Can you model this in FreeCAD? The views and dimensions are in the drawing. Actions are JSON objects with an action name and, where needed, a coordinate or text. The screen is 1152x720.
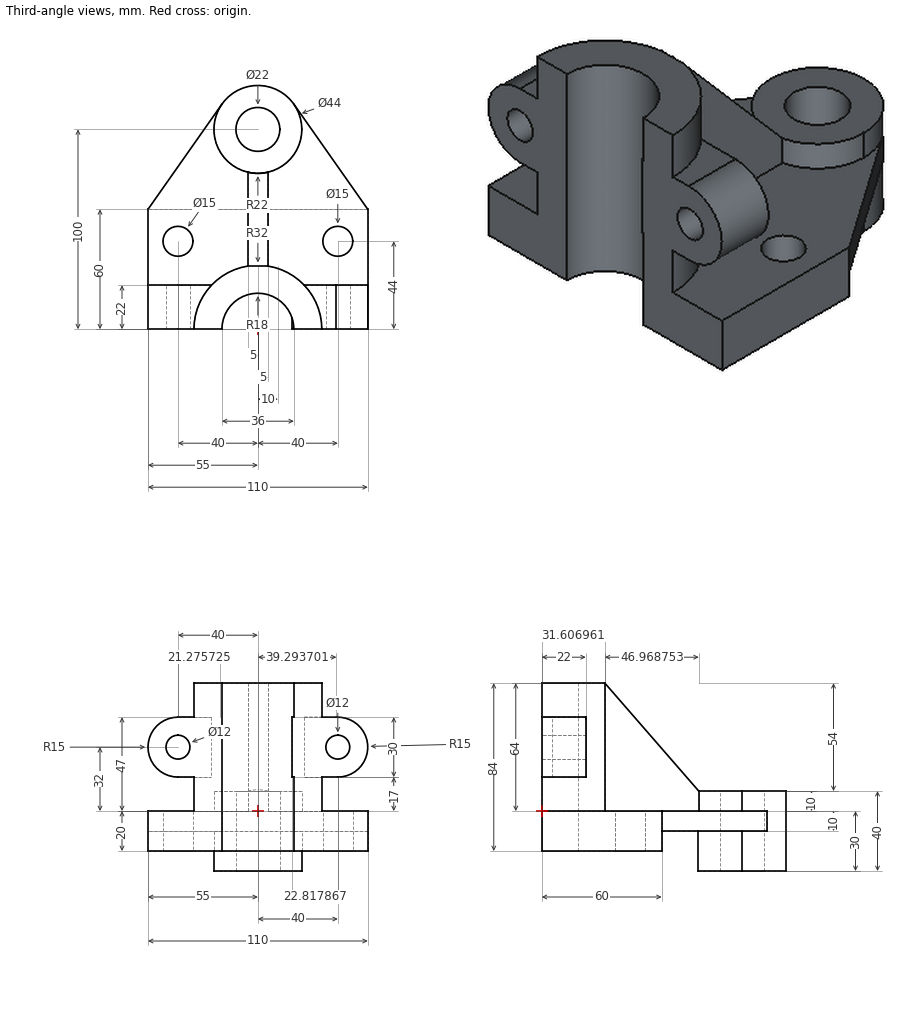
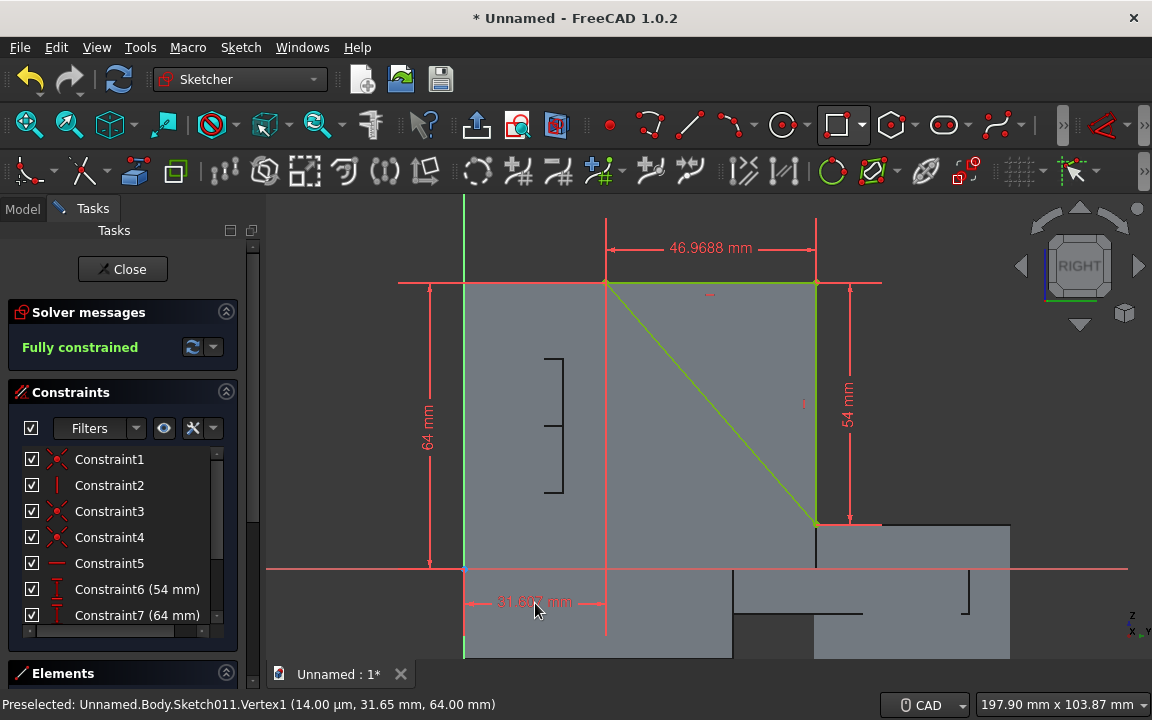
{"action": "left_click", "coordinate": [123, 269]}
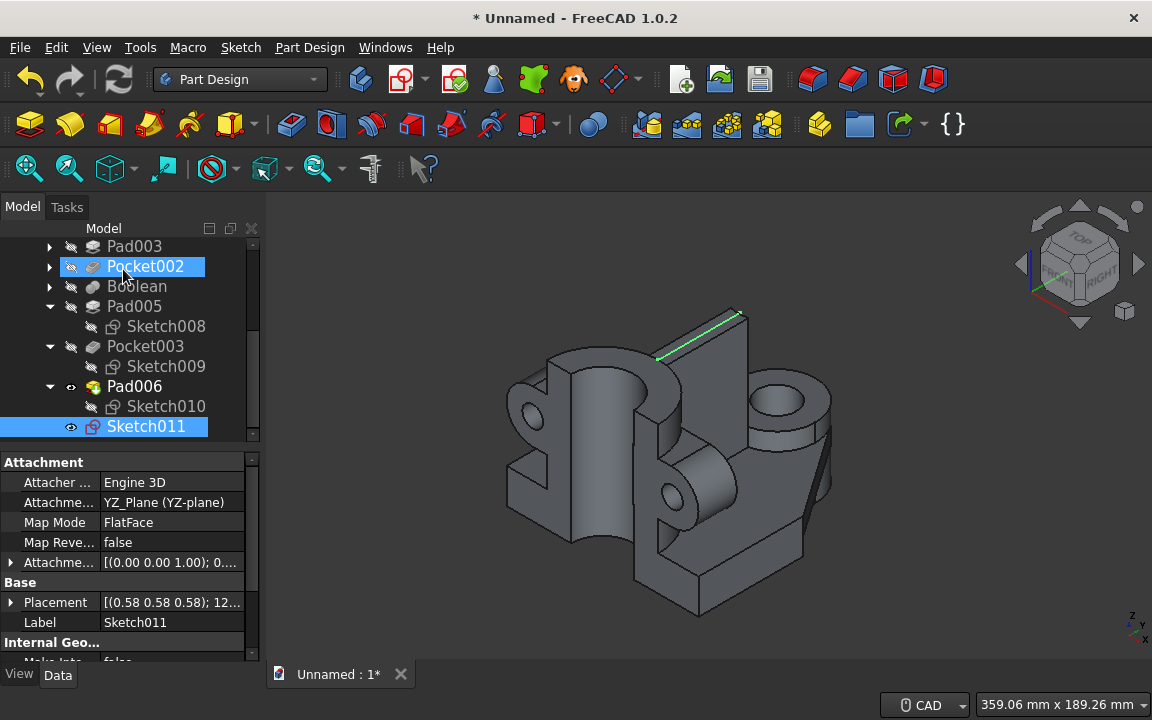
{"action": "left_click", "coordinate": [292, 124]}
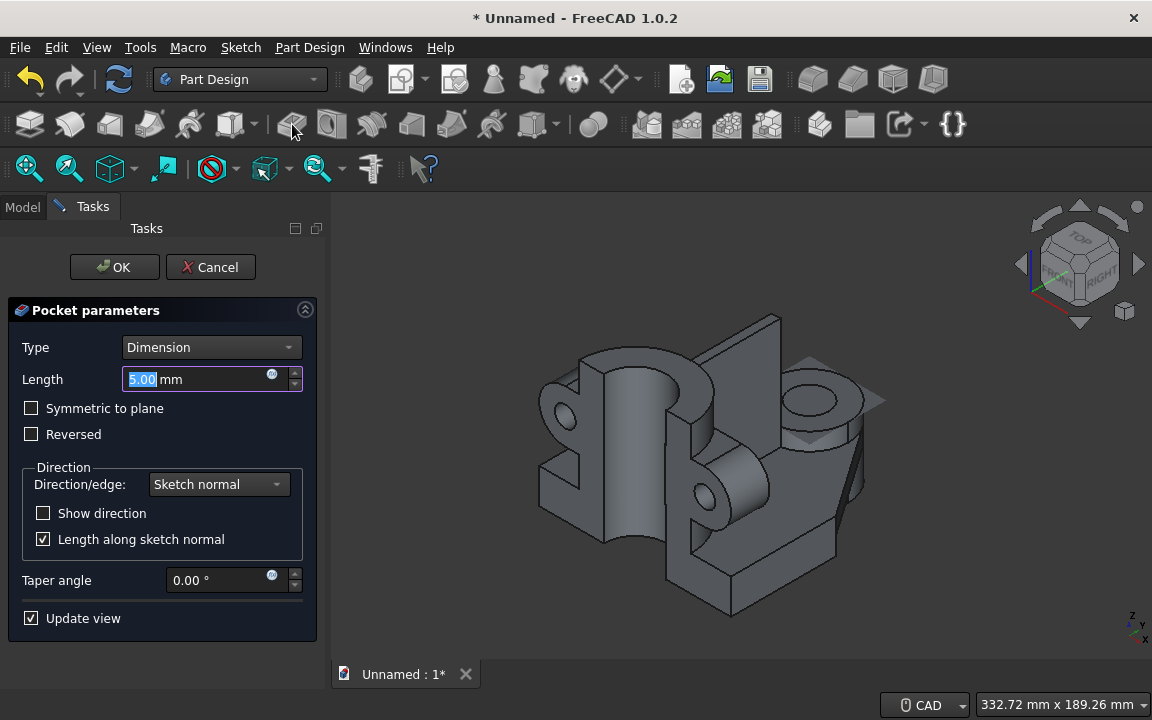
{"action": "type", "text": "64"}
{"action": "key", "text": "Tab"}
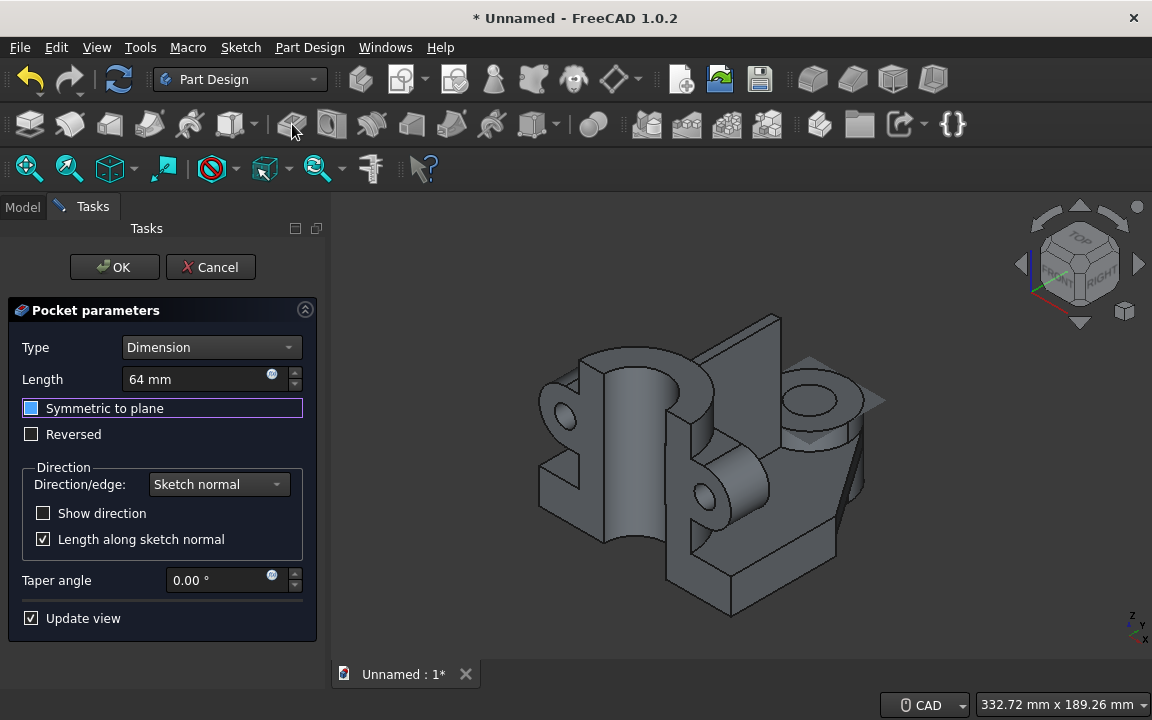
{"action": "left_click", "coordinate": [115, 267]}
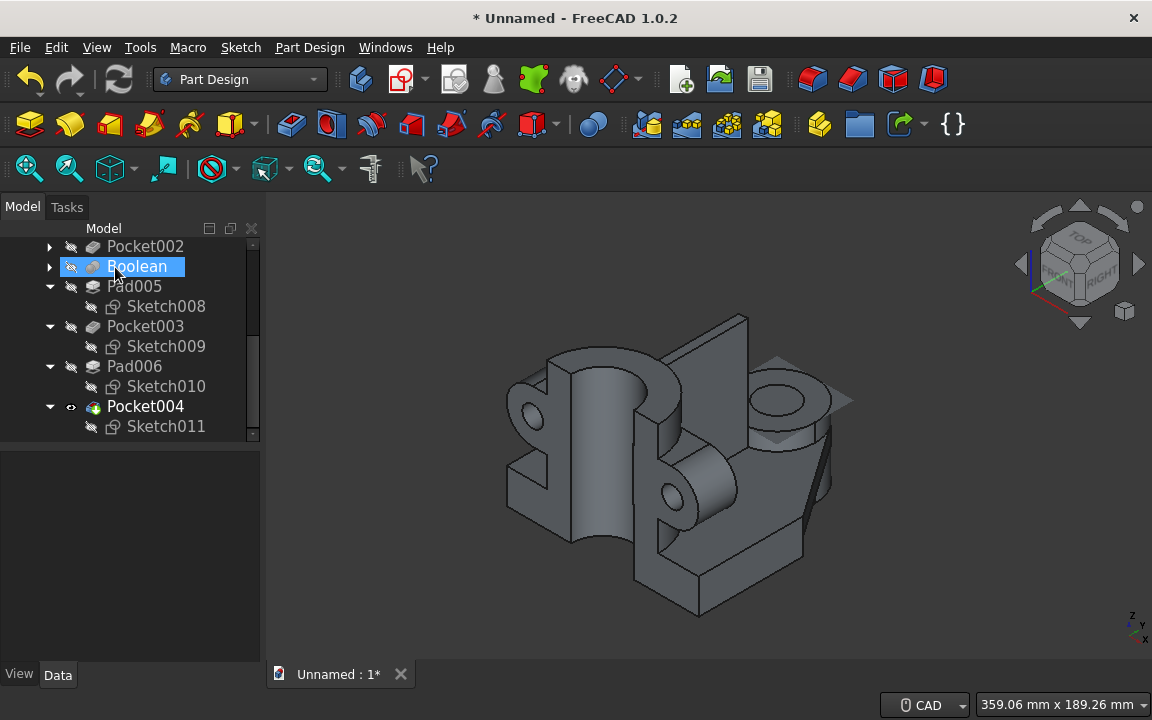
{"action": "key", "text": "6"}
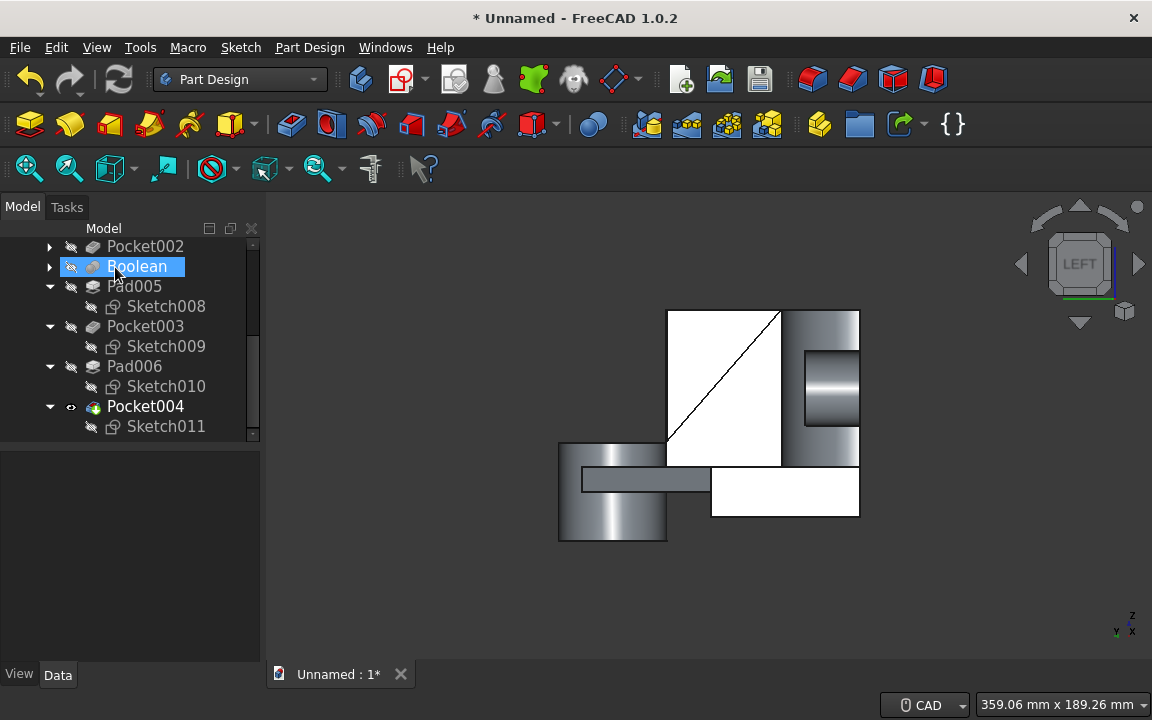
{"action": "left_click", "coordinate": [708, 337]}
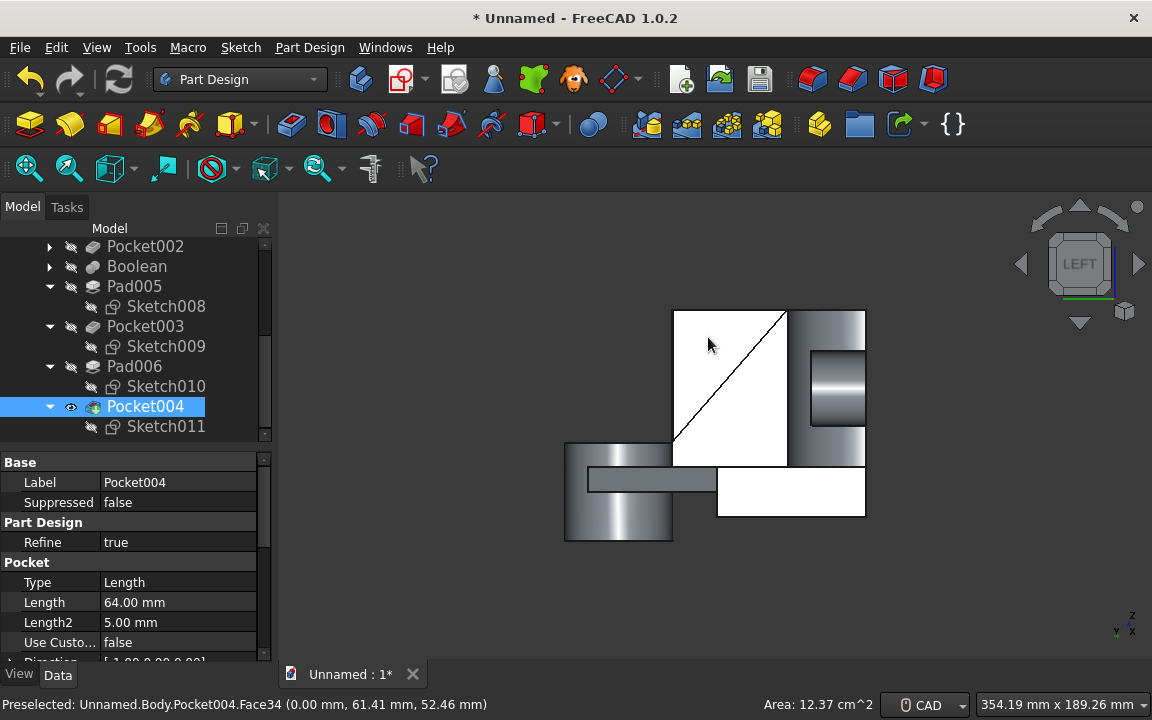
{"action": "left_click", "coordinate": [402, 80]}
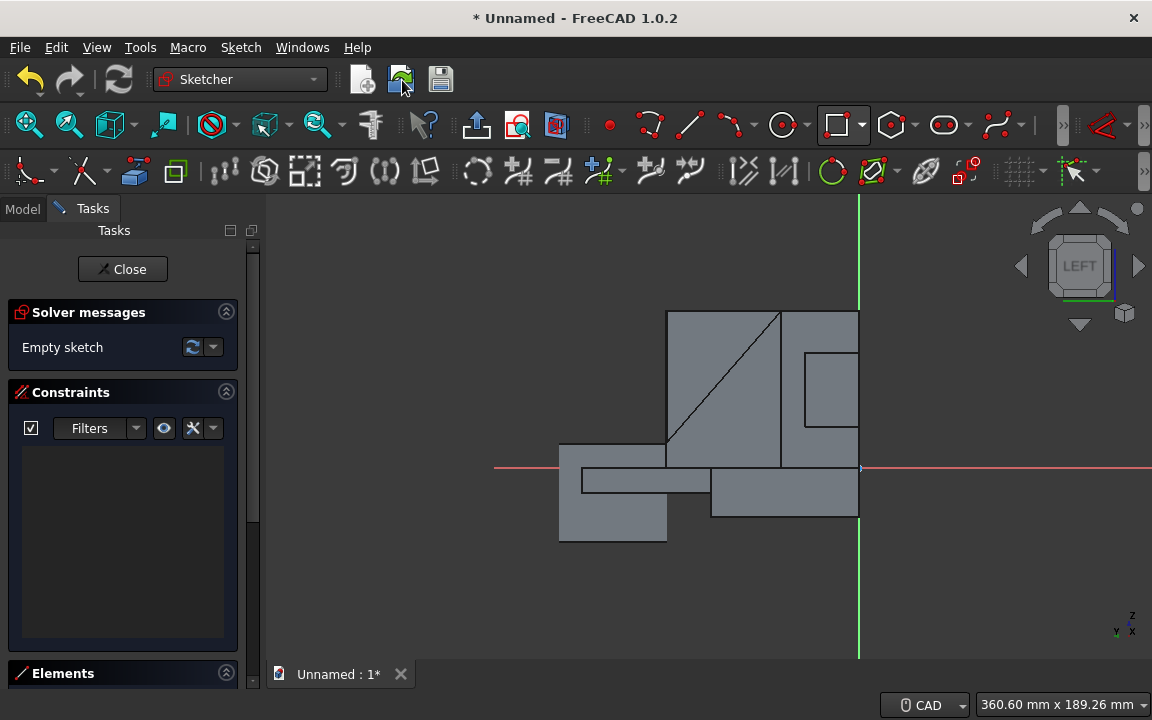
{"action": "scroll", "coordinate": [911, 345], "scroll_direction": "up", "scroll_amount": 3}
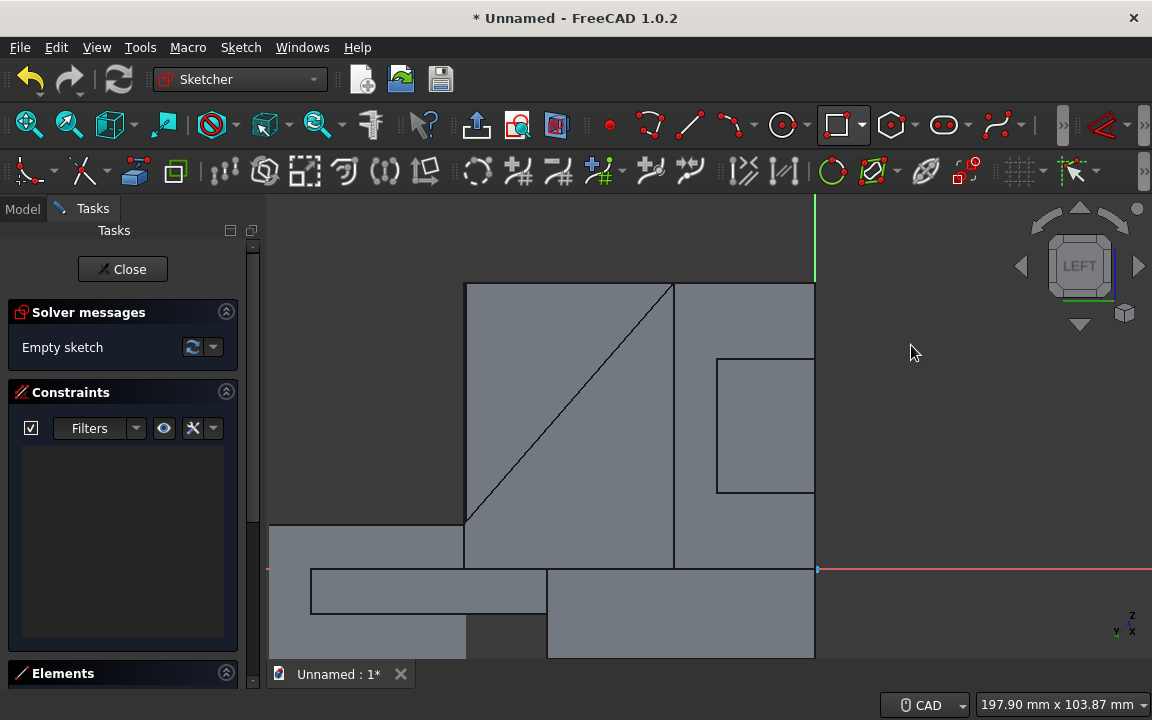
{"action": "left_click", "coordinate": [650, 126]}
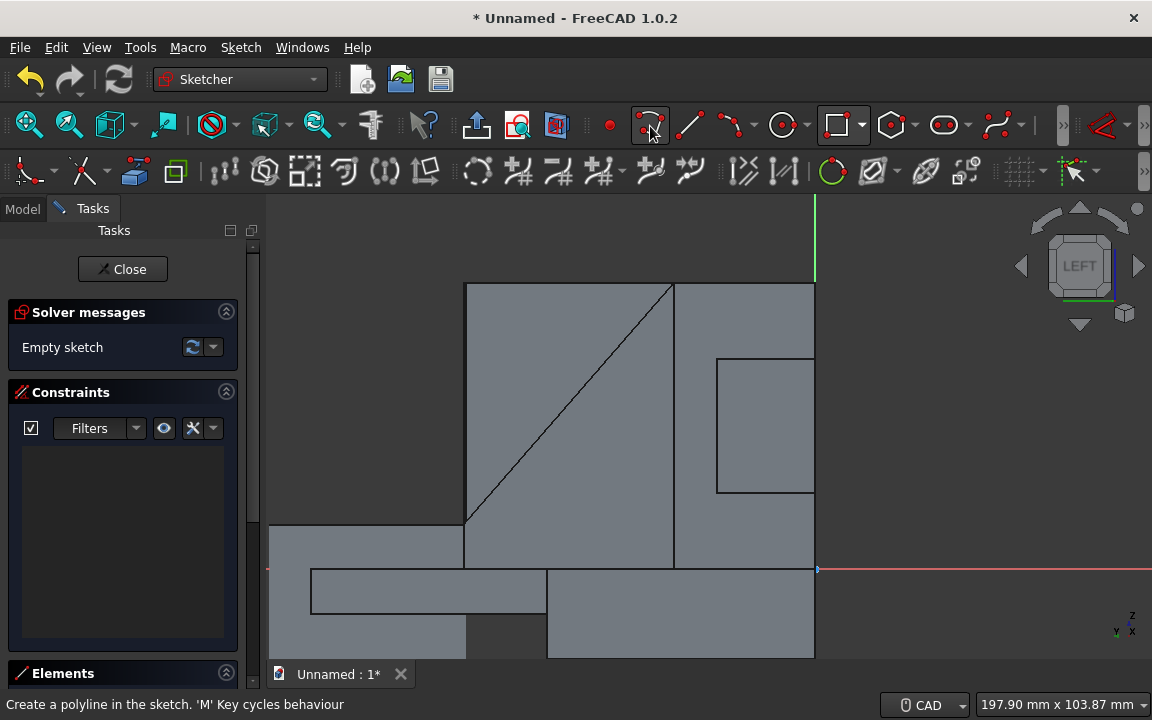
{"action": "left_click", "coordinate": [674, 283]}
{"action": "left_click", "coordinate": [464, 283]}
{"action": "left_click", "coordinate": [464, 525]}
{"action": "left_click", "coordinate": [674, 284]}
{"action": "key", "text": "Escape"}
{"action": "key", "text": "Escape"}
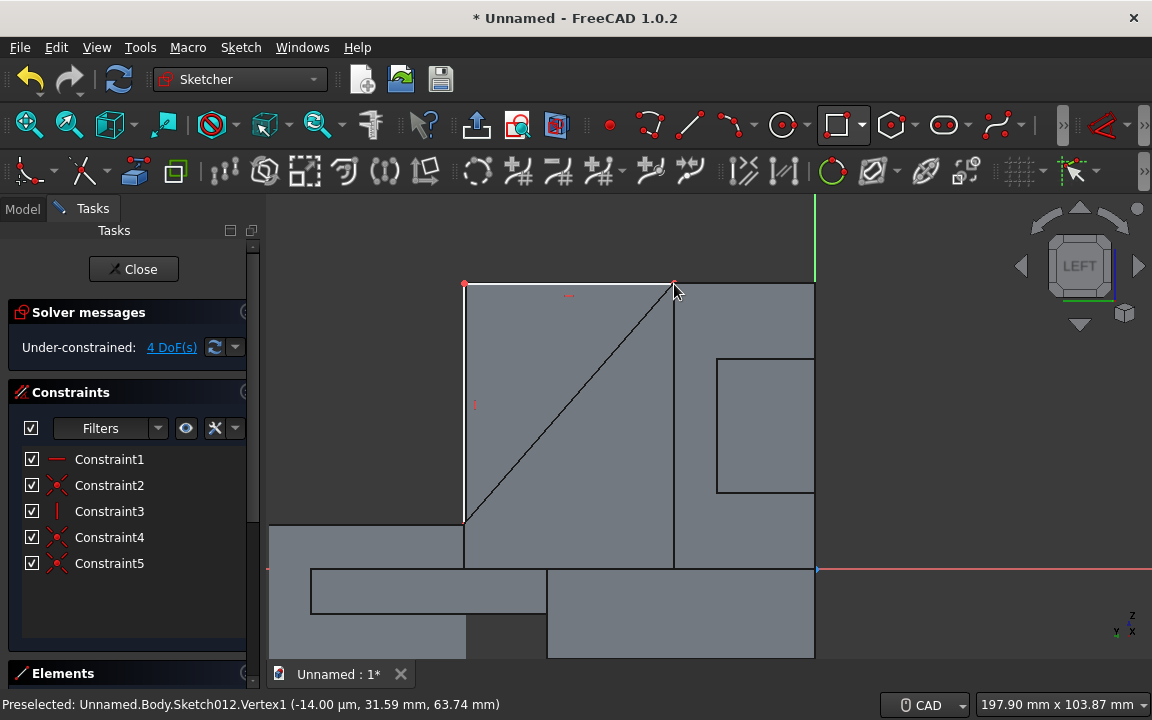
{"action": "left_click", "coordinate": [1102, 126]}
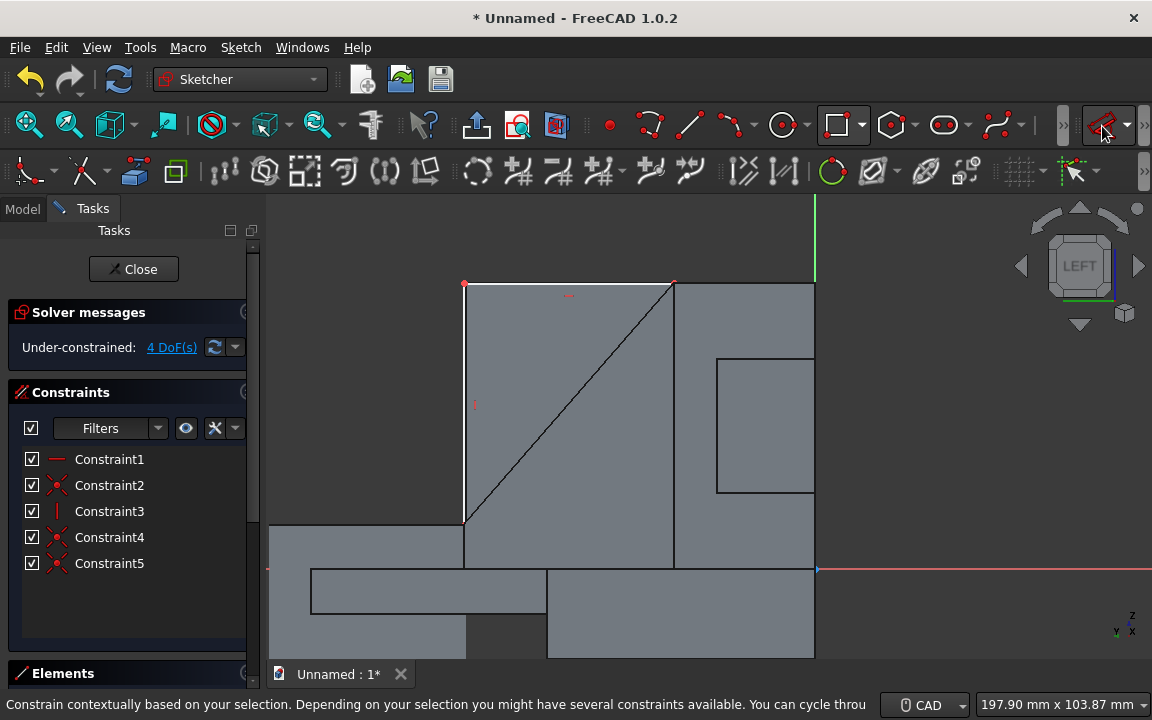
{"action": "left_click", "coordinate": [464, 357]}
{"action": "left_click", "coordinate": [430, 405]}